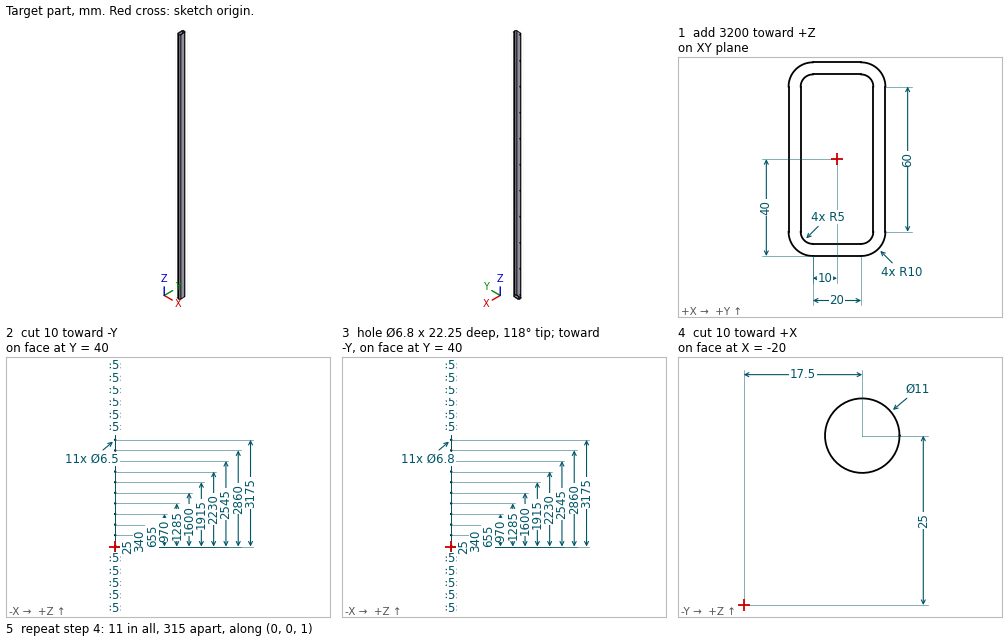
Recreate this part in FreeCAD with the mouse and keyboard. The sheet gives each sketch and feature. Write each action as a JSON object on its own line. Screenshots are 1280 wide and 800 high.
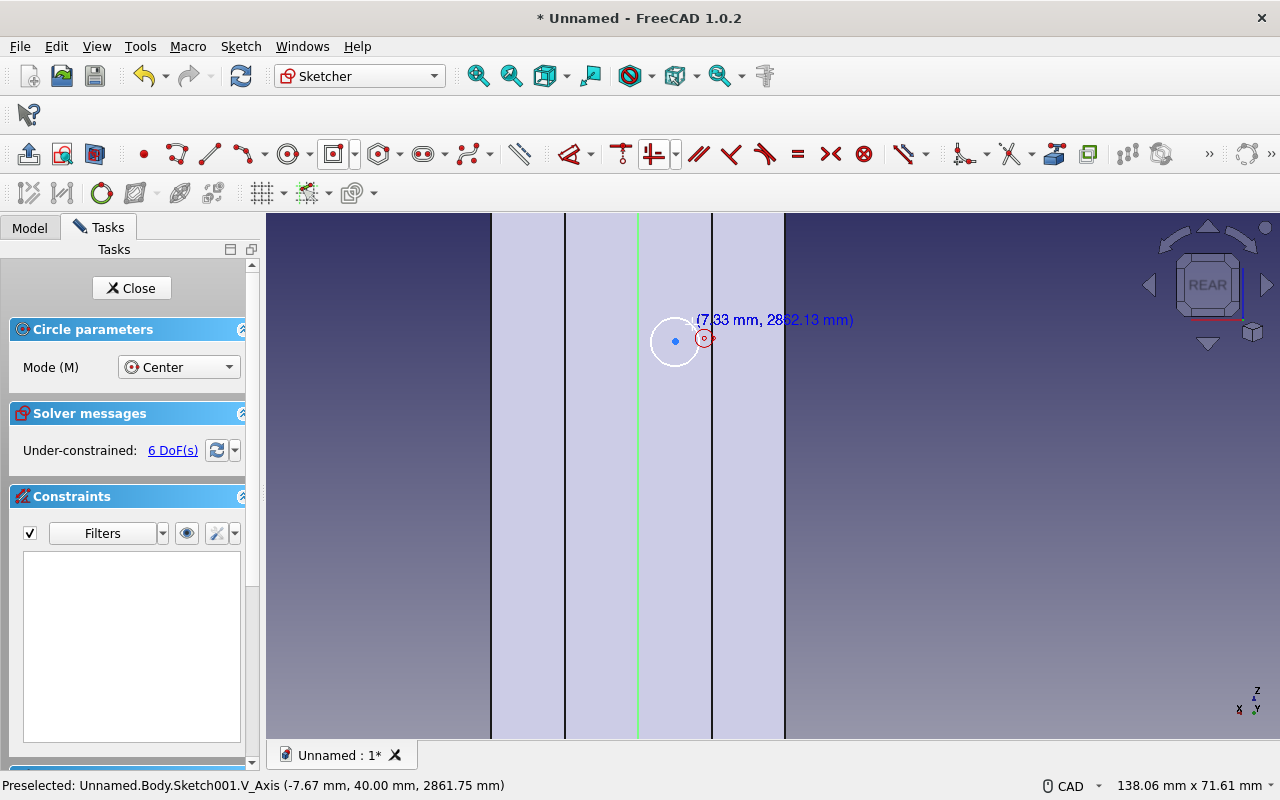
{"action": "scroll", "coordinate": [704, 476], "scroll_direction": "down", "scroll_amount": 15}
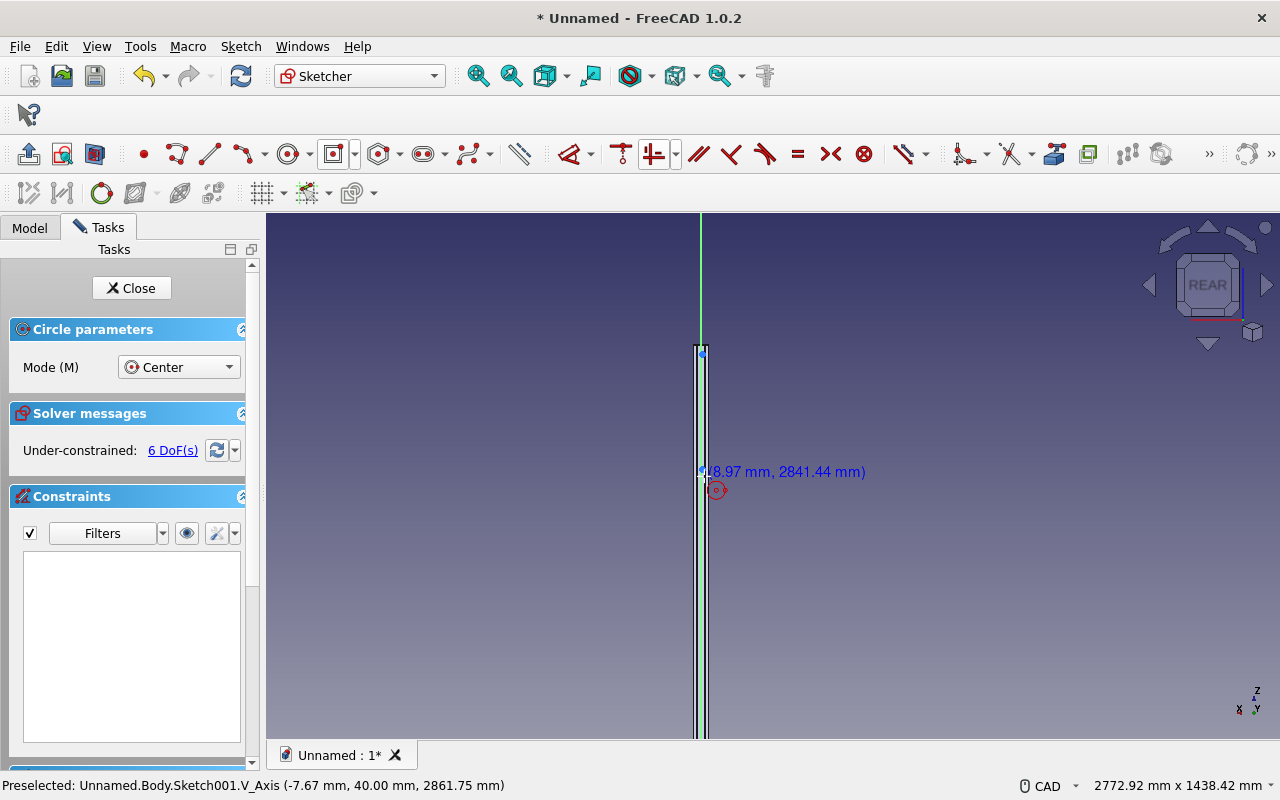
{"action": "scroll", "coordinate": [705, 278], "scroll_direction": "down", "scroll_amount": 6}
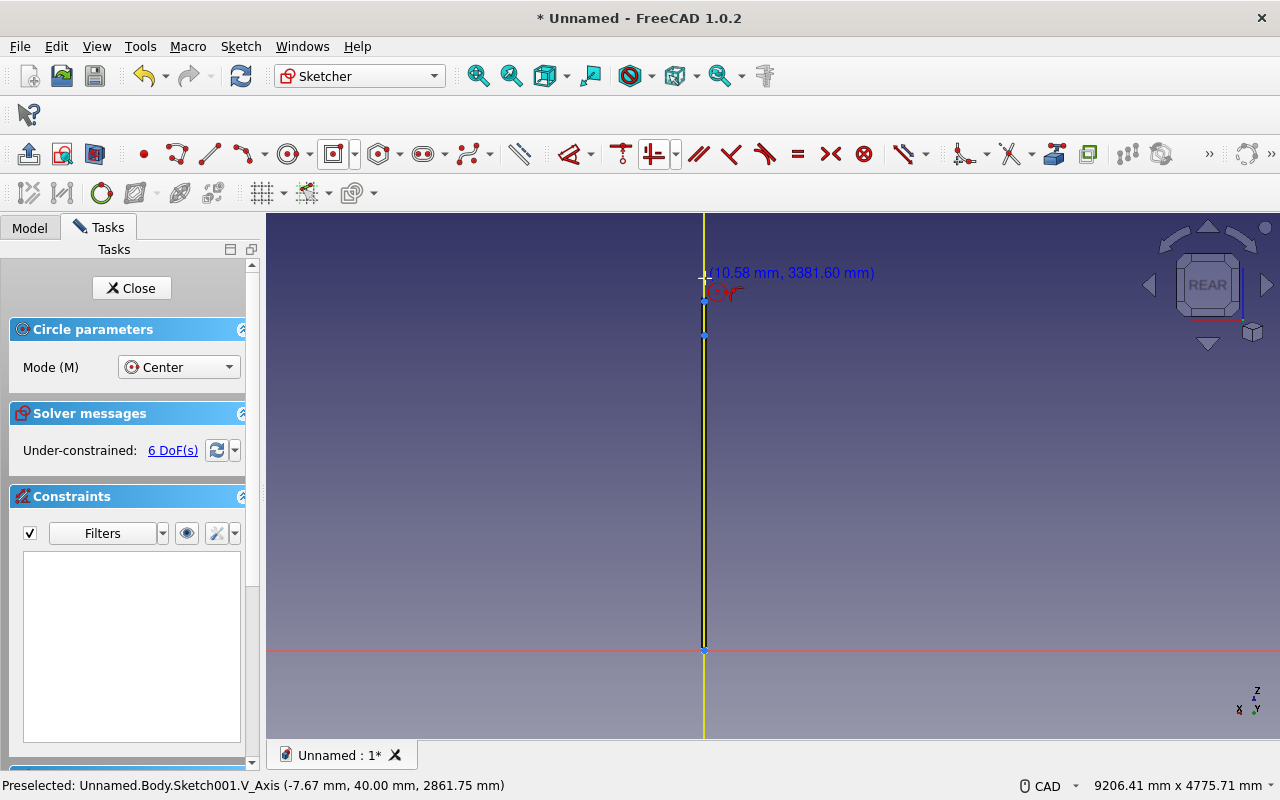
{"action": "scroll", "coordinate": [705, 371], "scroll_direction": "up", "scroll_amount": 21}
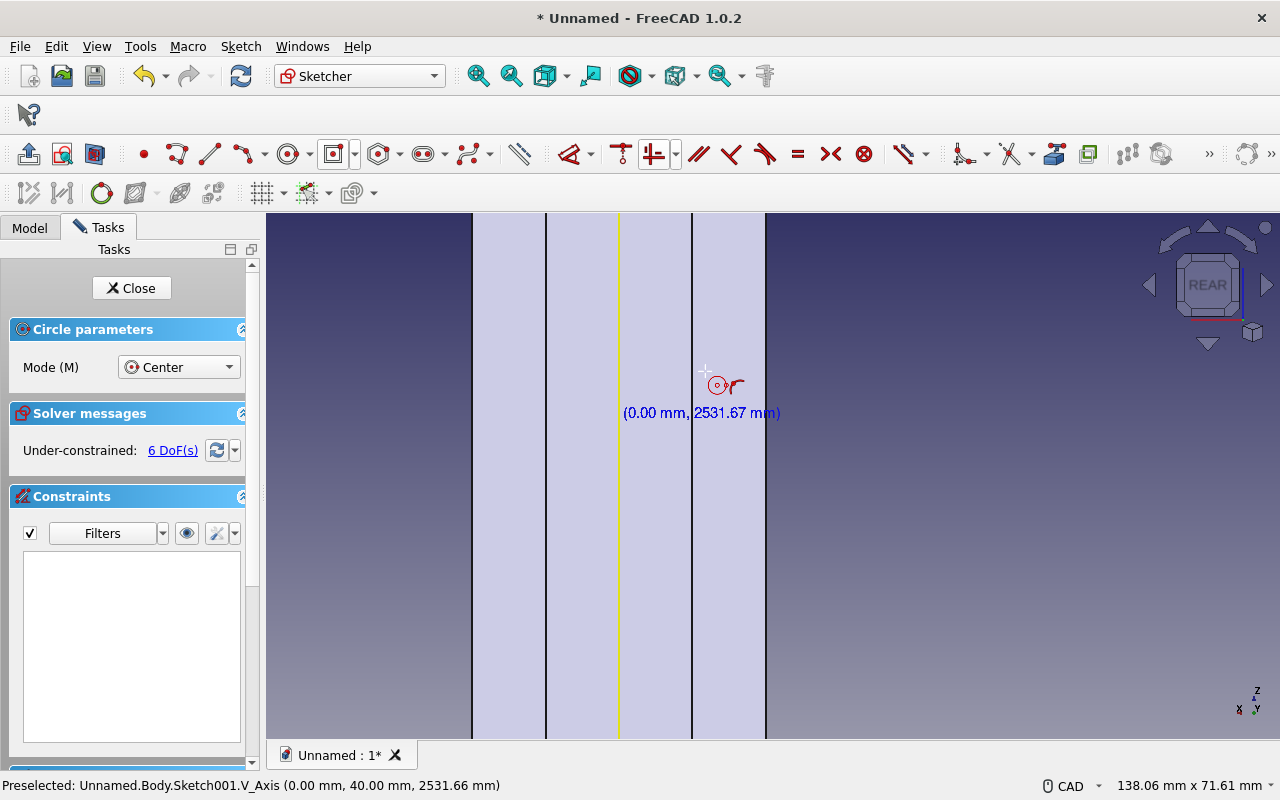
{"action": "left_click", "coordinate": [656, 320]}
{"action": "left_click", "coordinate": [673, 303]}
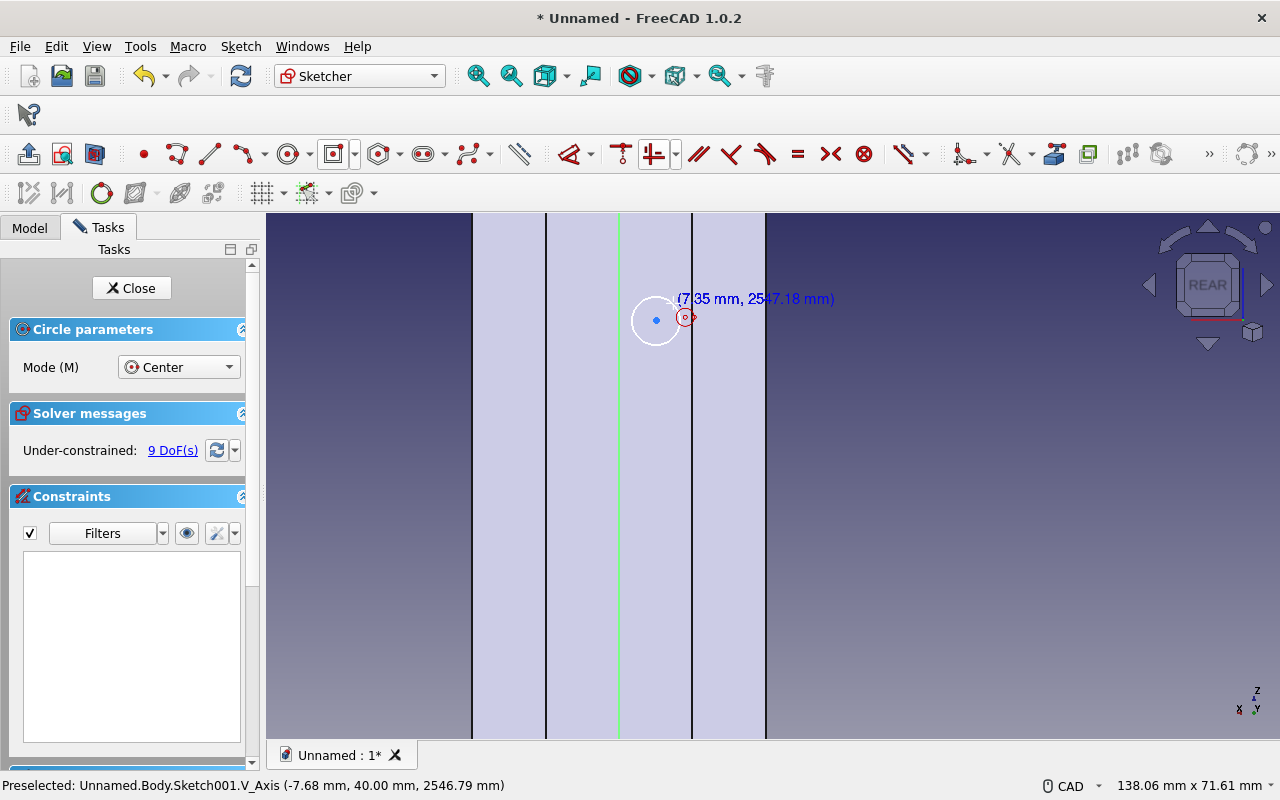
{"action": "scroll", "coordinate": [704, 476], "scroll_direction": "down", "scroll_amount": 15}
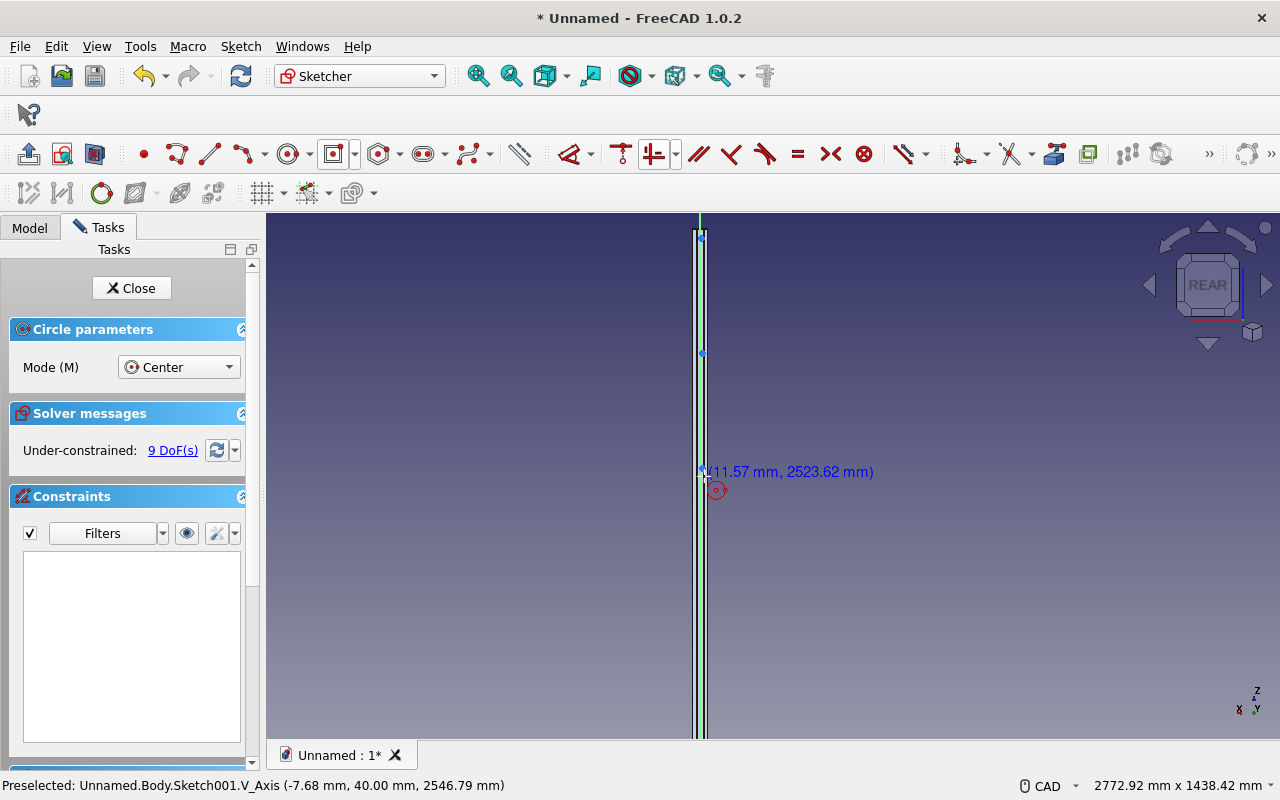
{"action": "scroll", "coordinate": [706, 328], "scroll_direction": "down", "scroll_amount": 6}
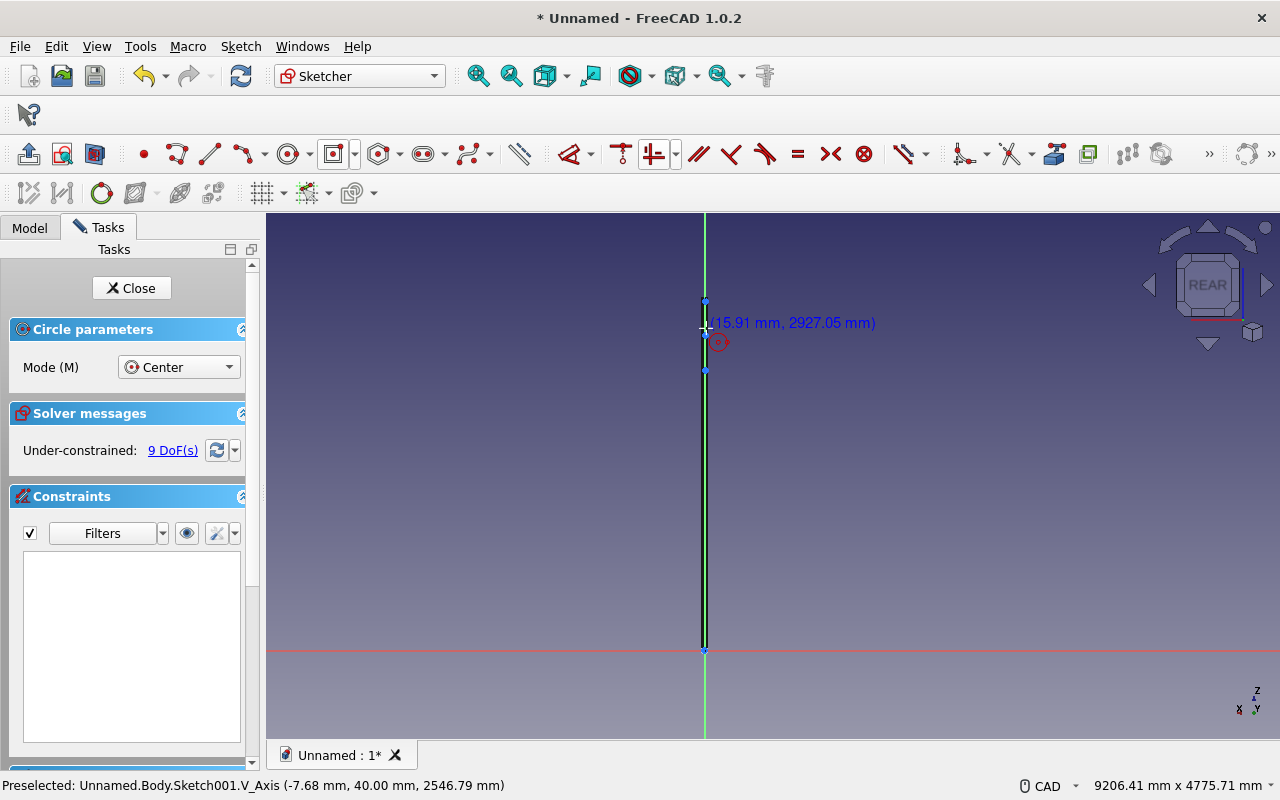
{"action": "scroll", "coordinate": [705, 405], "scroll_direction": "up", "scroll_amount": 21}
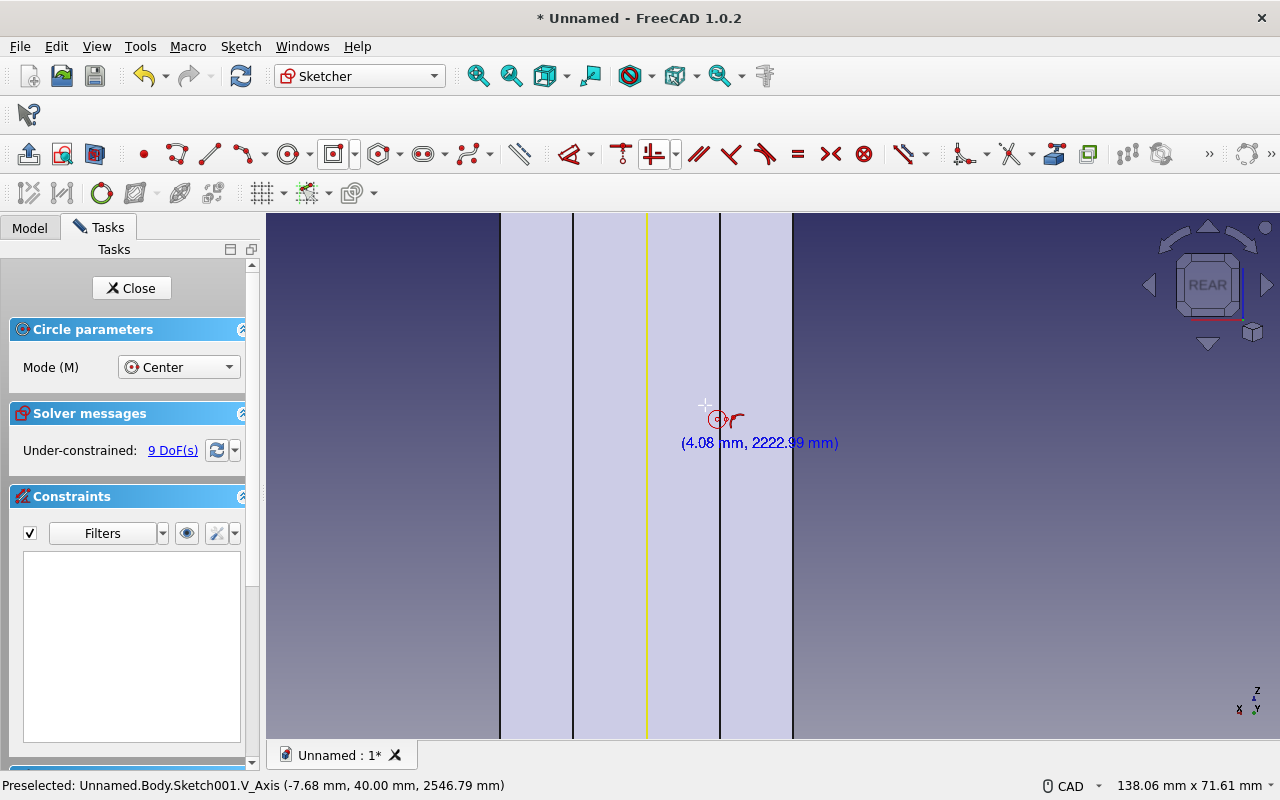
{"action": "left_click", "coordinate": [683, 396]}
{"action": "left_click", "coordinate": [700, 379]}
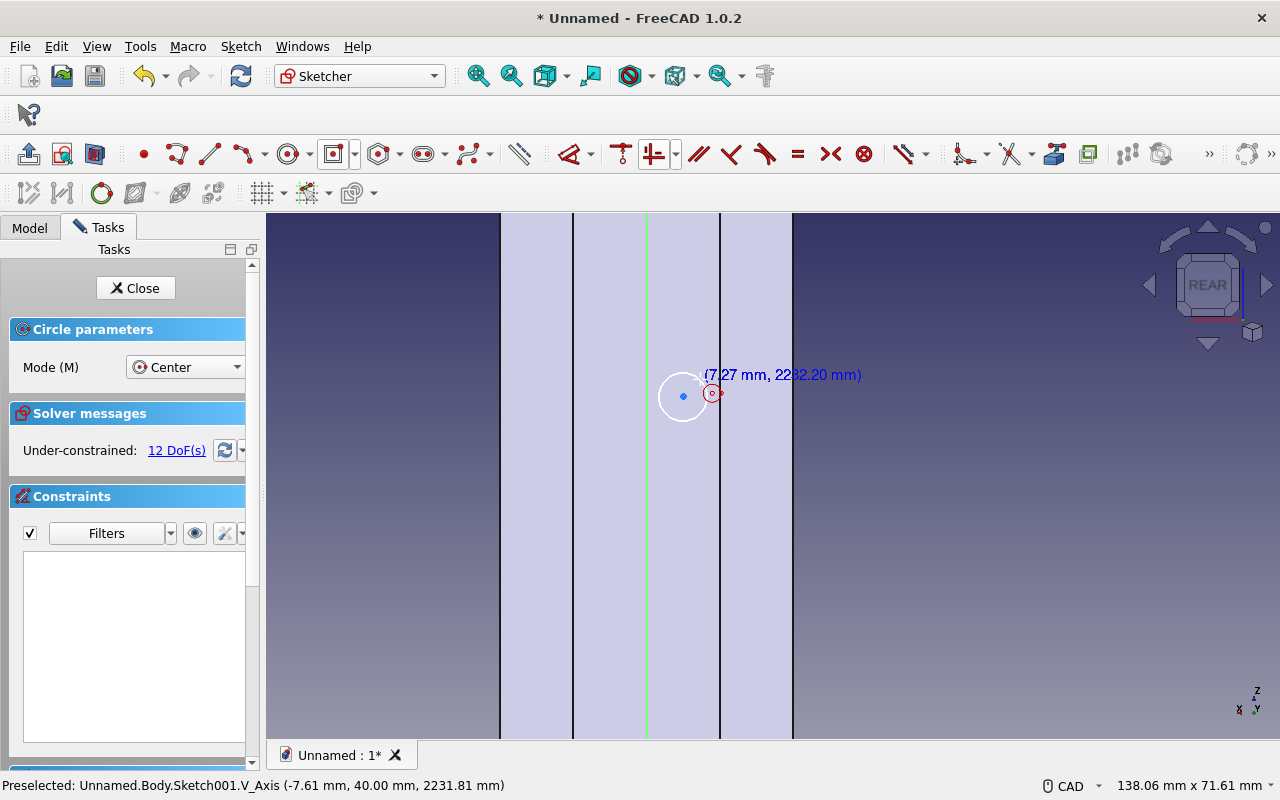
{"action": "scroll", "coordinate": [704, 476], "scroll_direction": "down", "scroll_amount": 15}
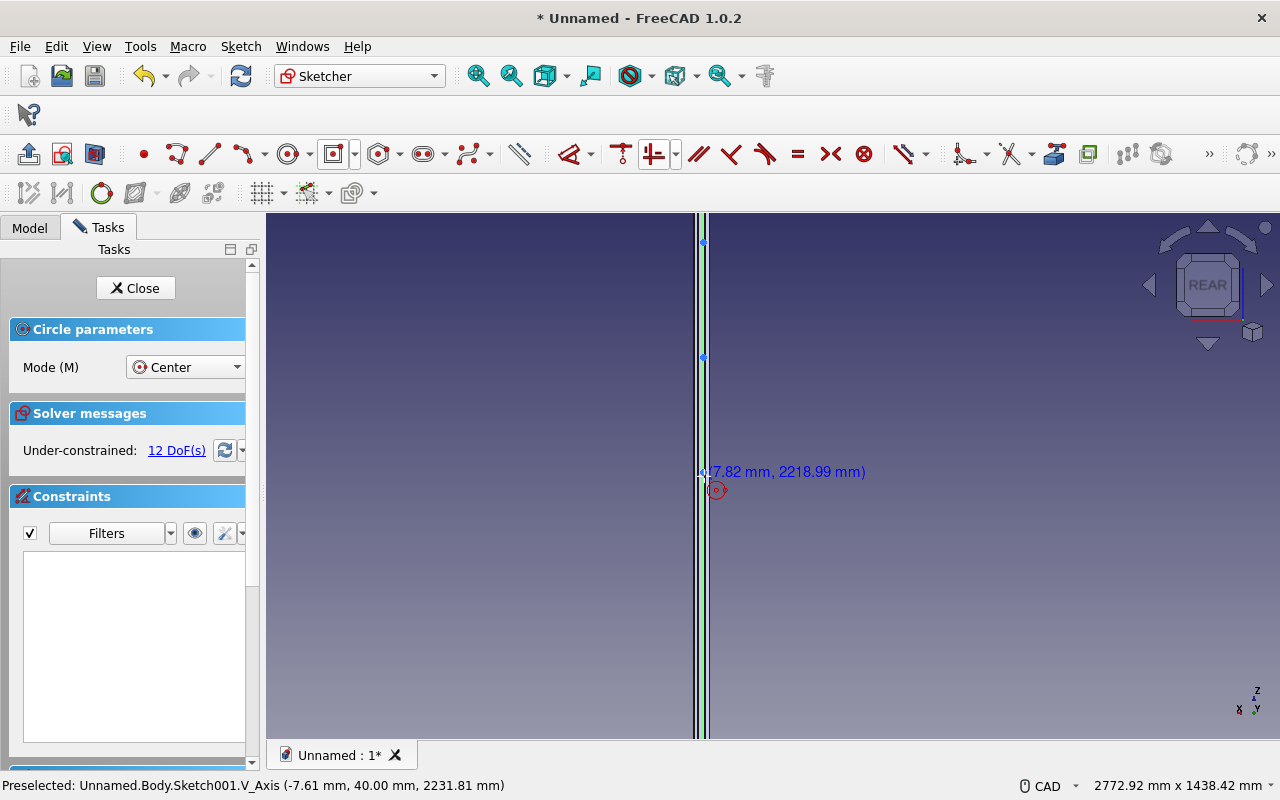
{"action": "scroll", "coordinate": [705, 376], "scroll_direction": "down", "scroll_amount": 6}